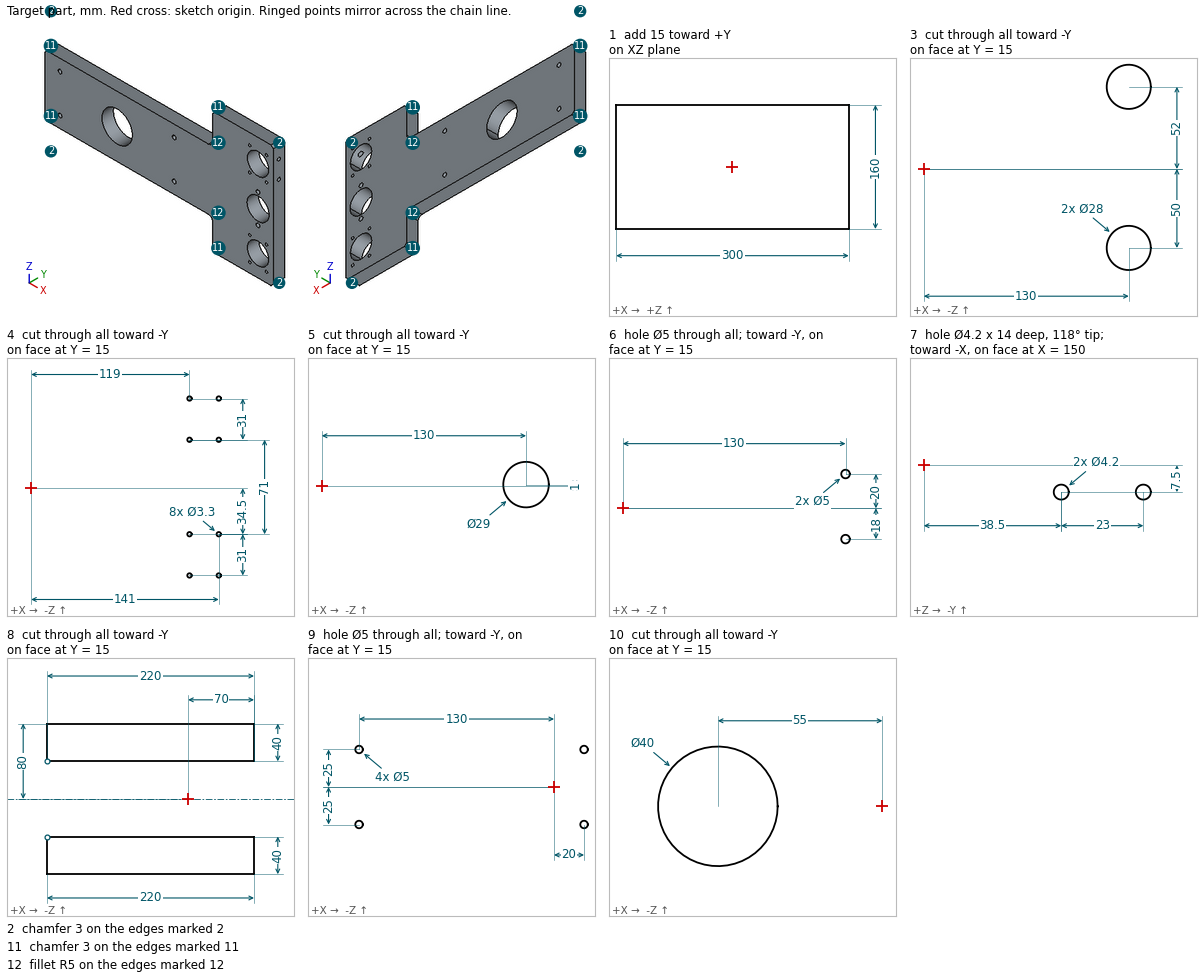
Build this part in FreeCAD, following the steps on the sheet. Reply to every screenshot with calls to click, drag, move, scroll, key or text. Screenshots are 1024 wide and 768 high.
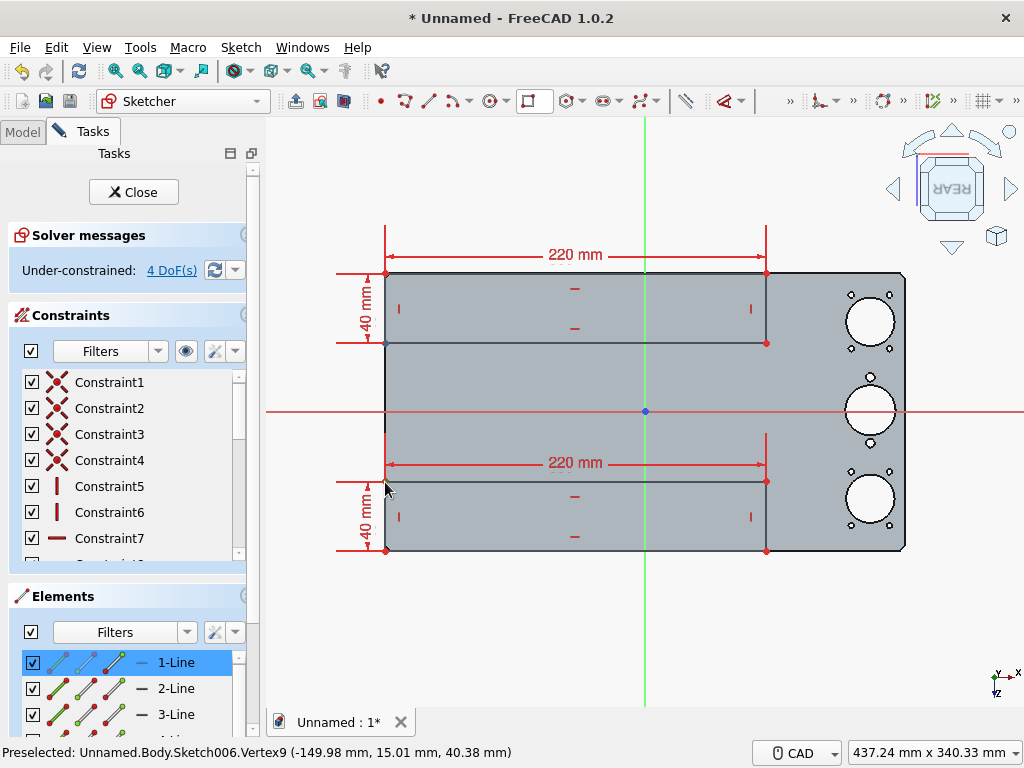
click(334, 412)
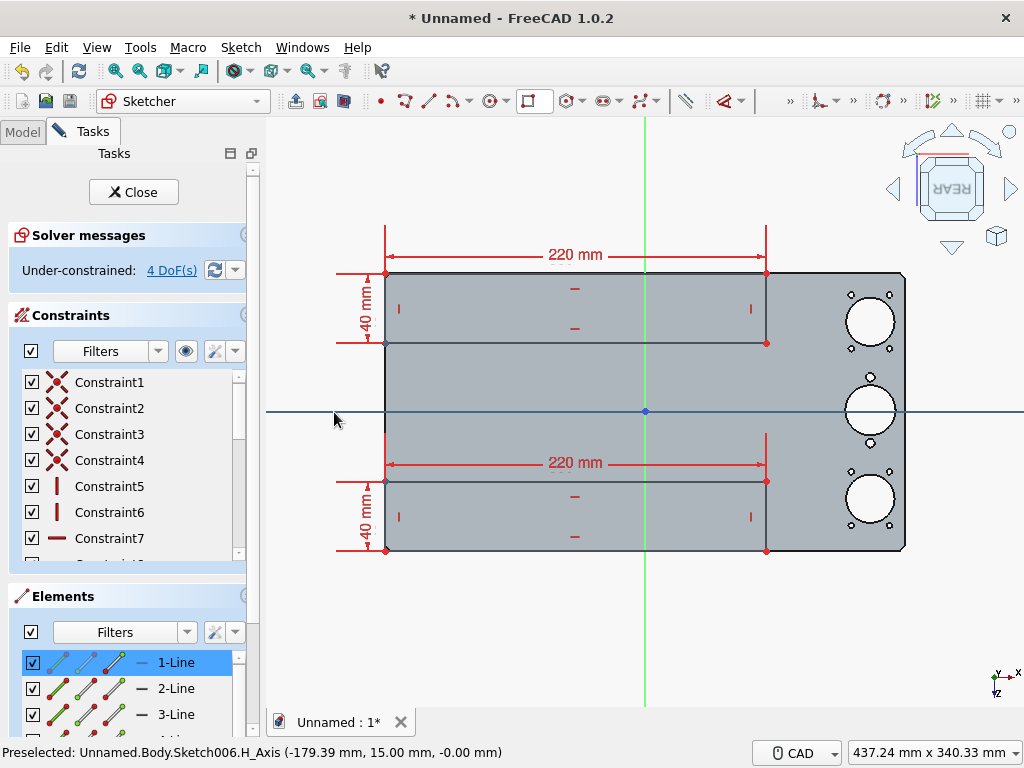
key(s)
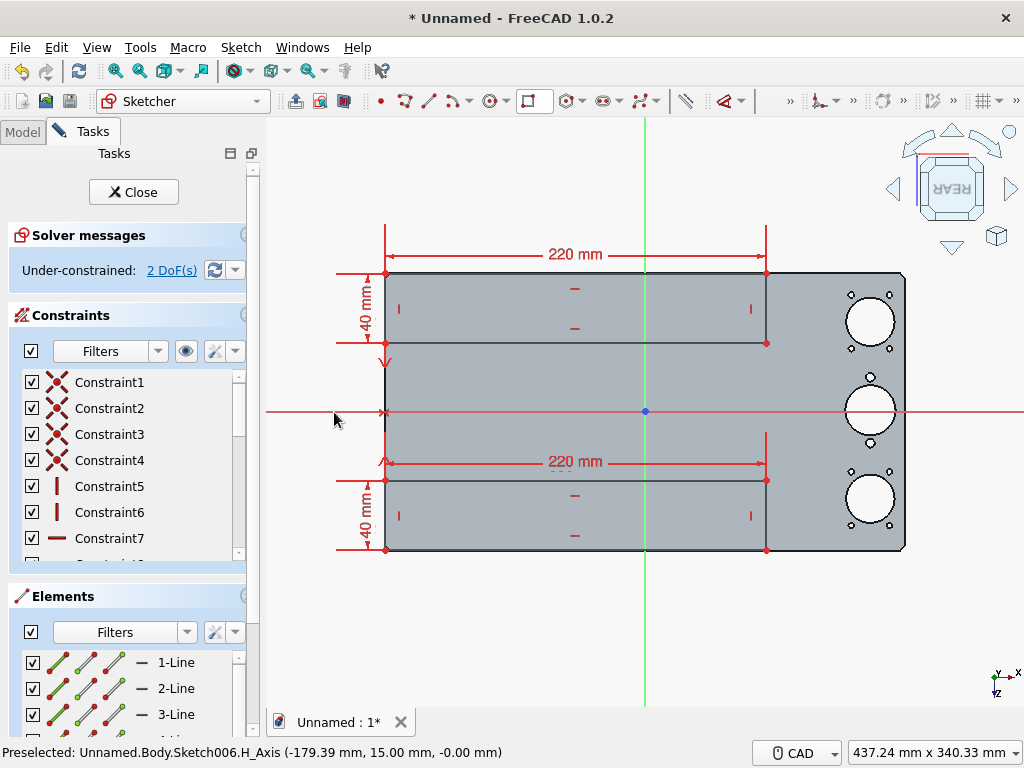
click(724, 102)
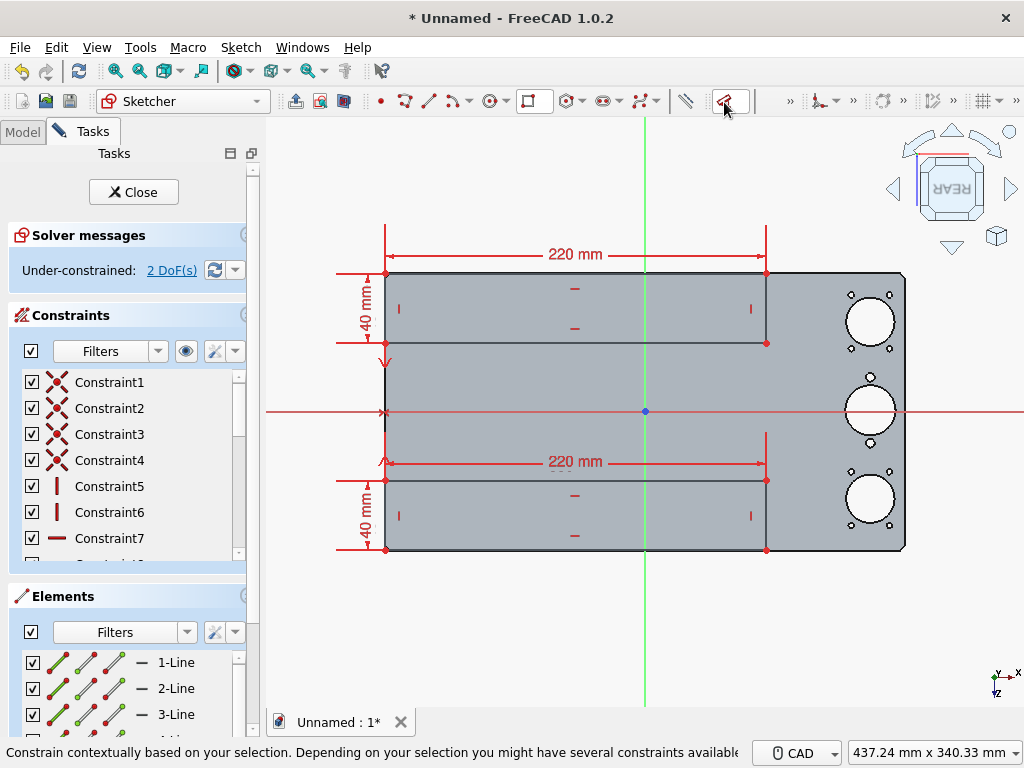
click(385, 274)
click(351, 343)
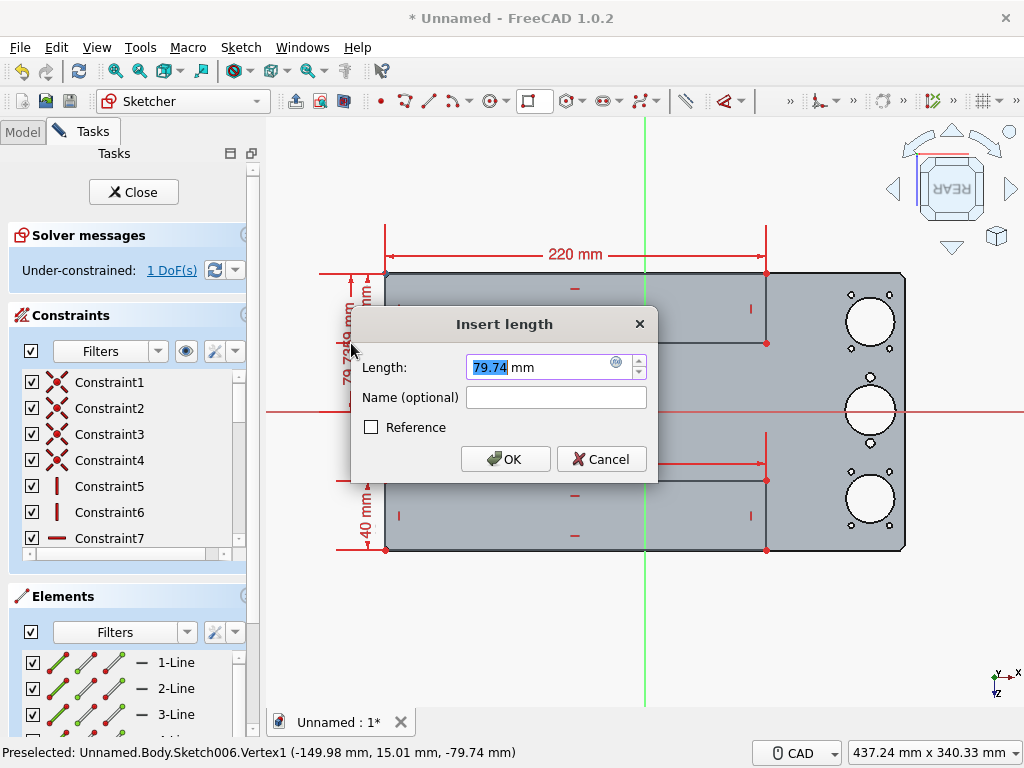
text(80)
key(Return)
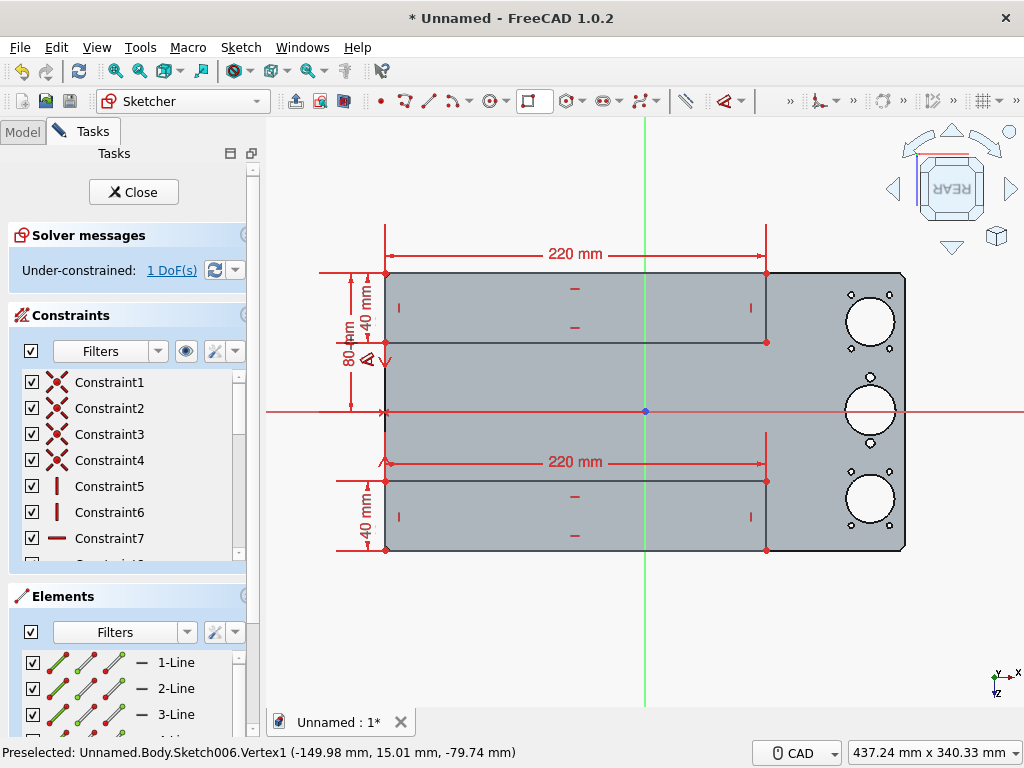
click(766, 343)
click(706, 309)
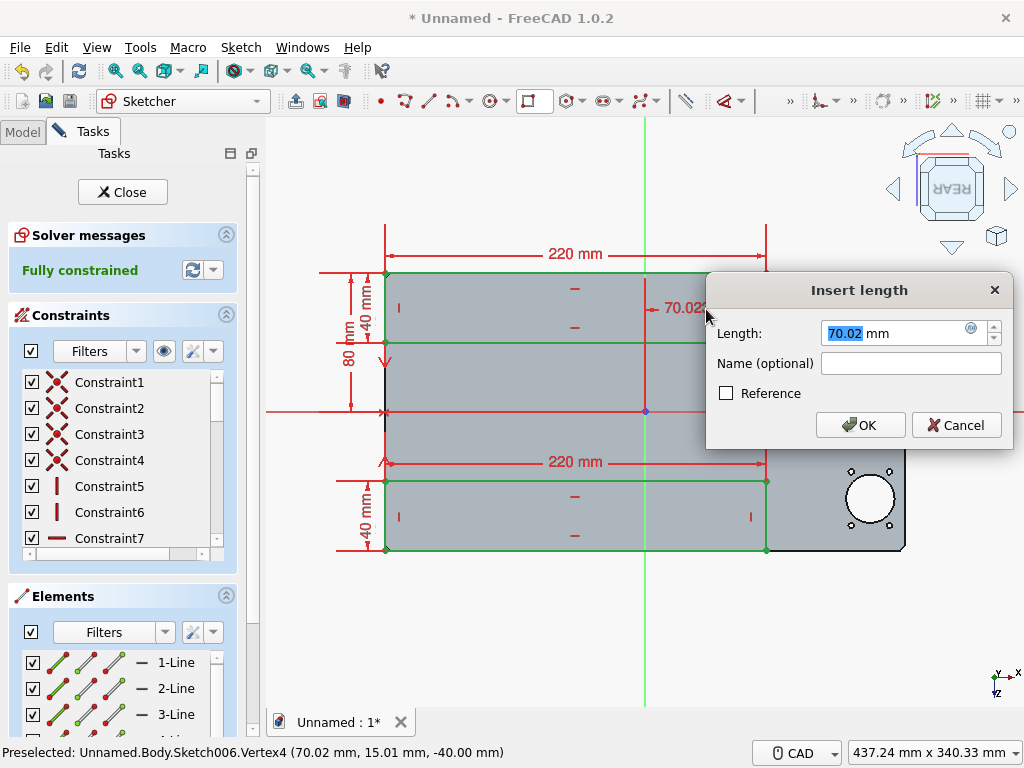
text(70)
key(Return)
key(Escape)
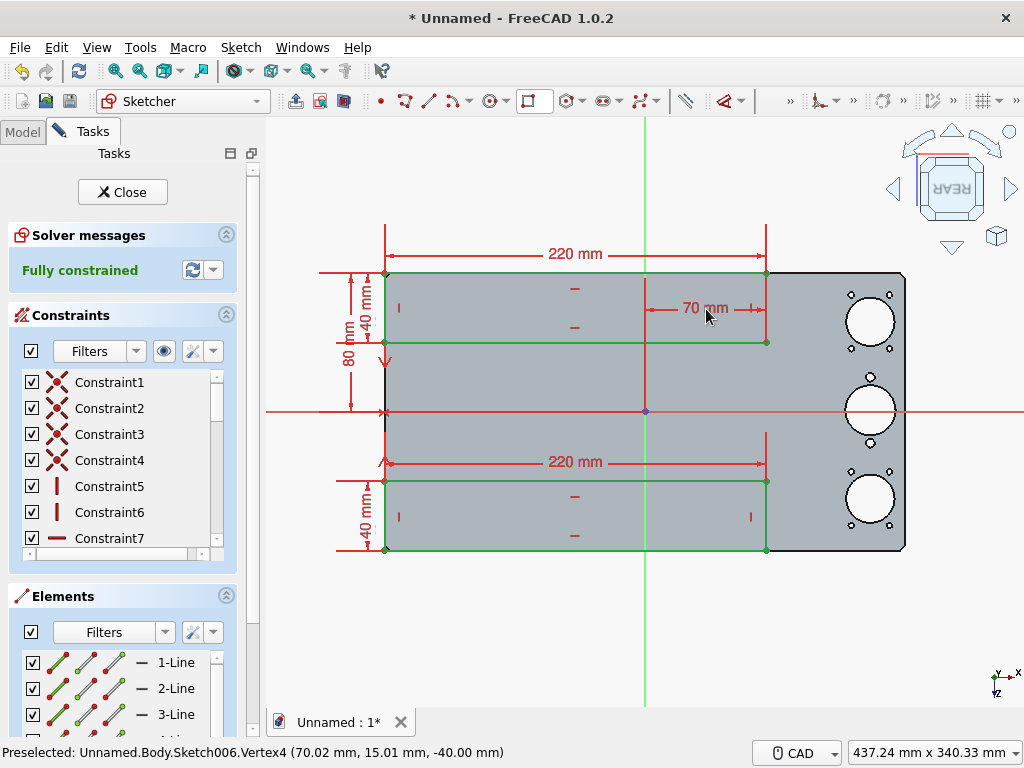
click(123, 192)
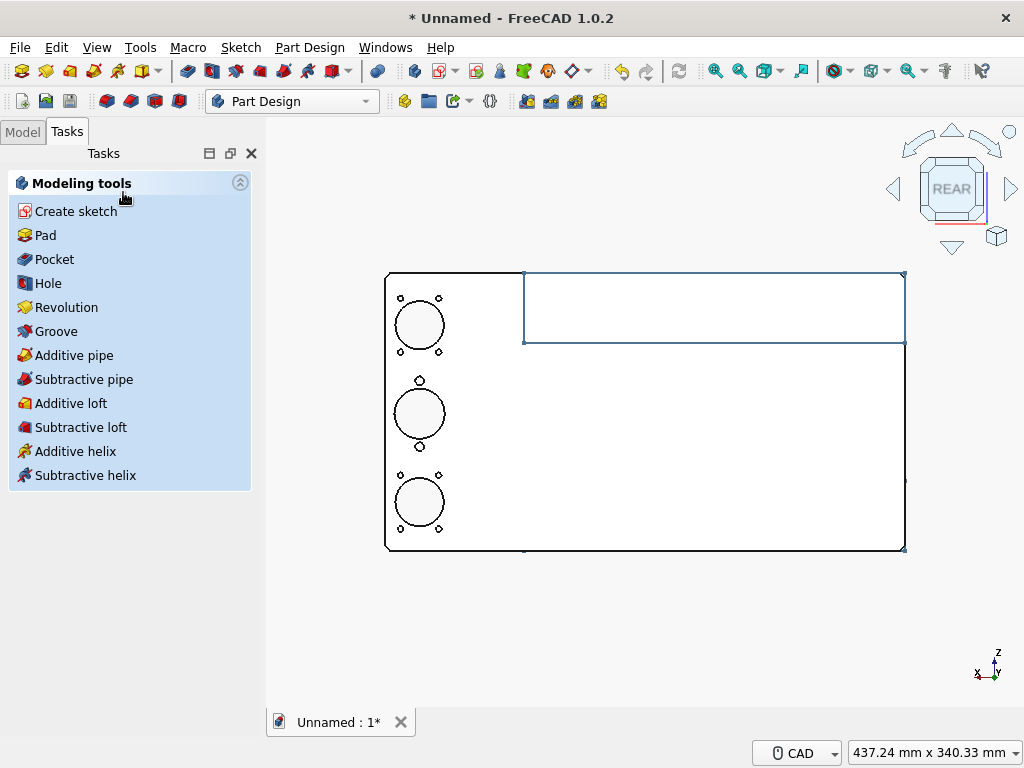
click(188, 72)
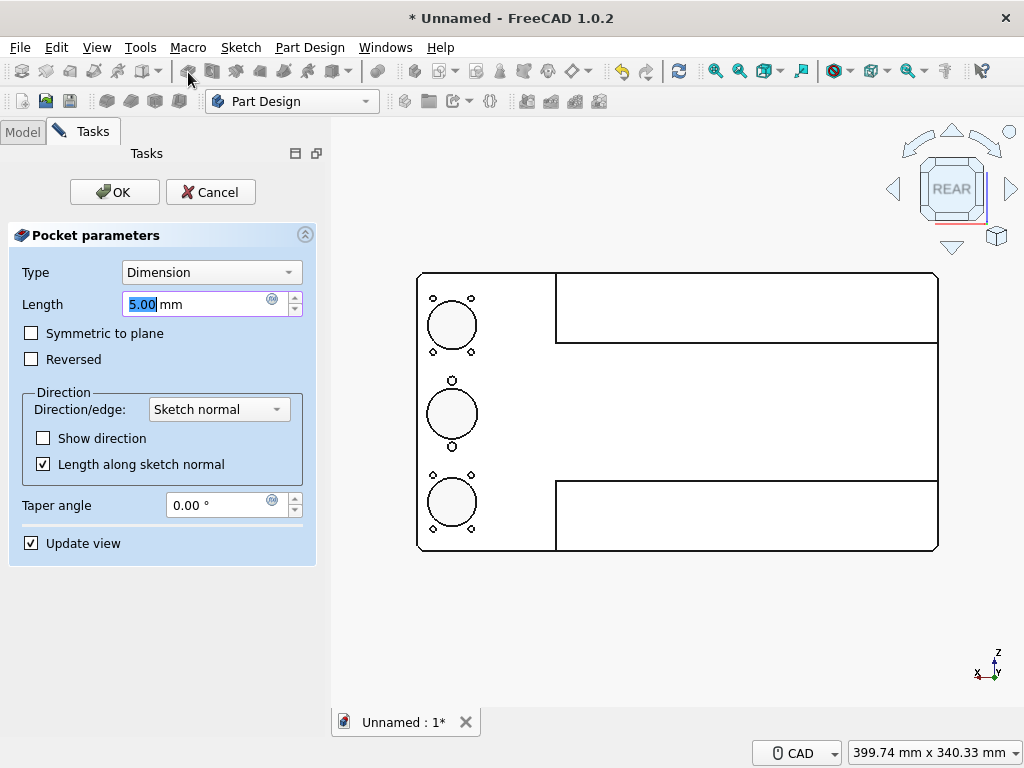
click(212, 272)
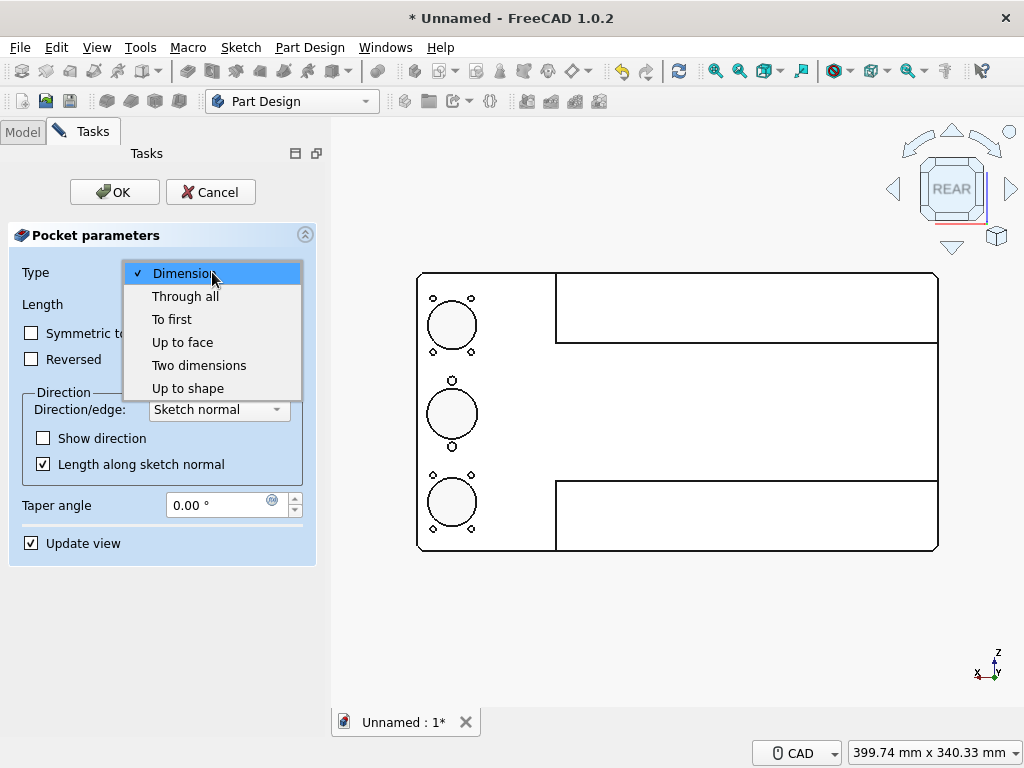
click(212, 296)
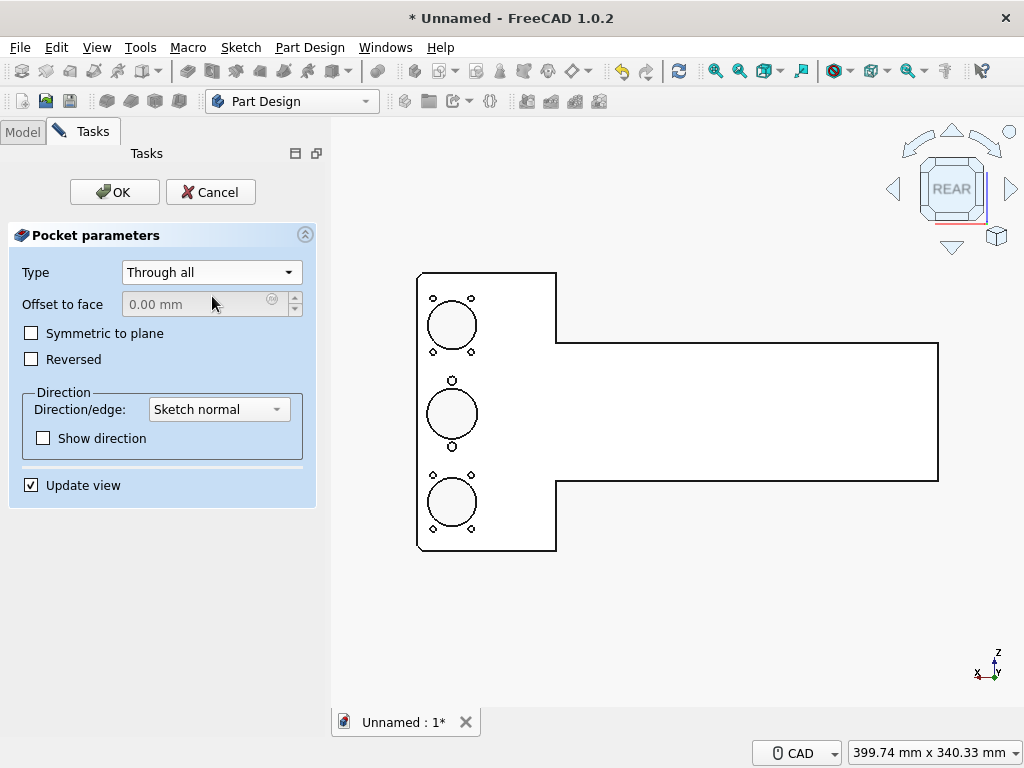
click(115, 192)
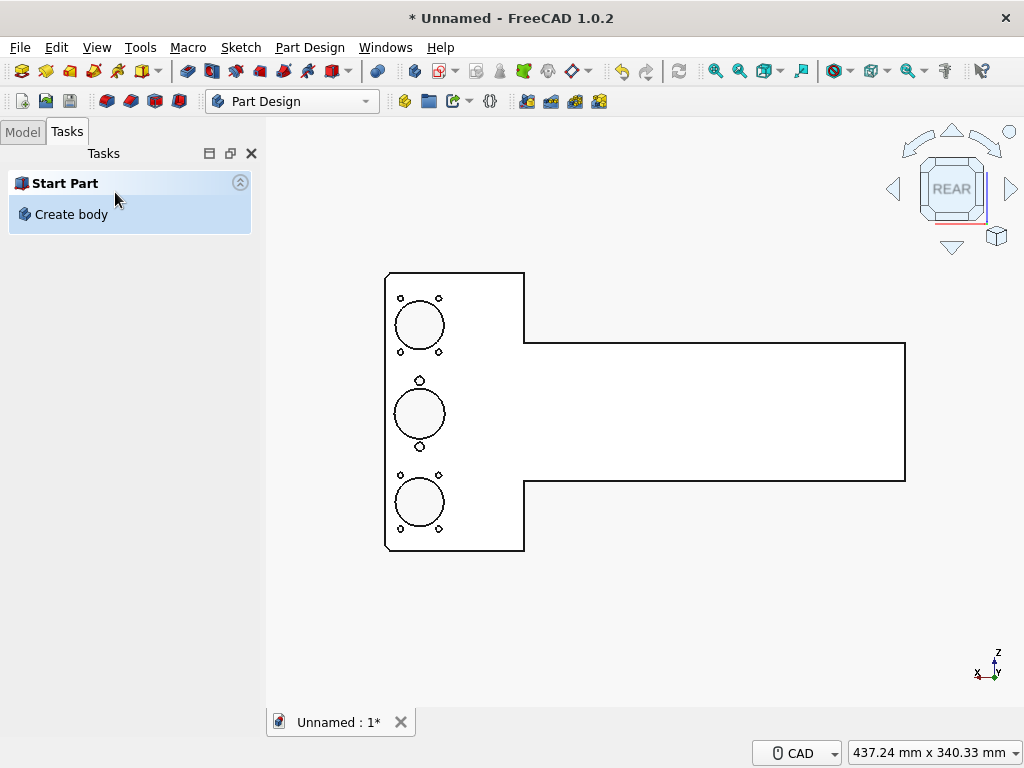
click(571, 411)